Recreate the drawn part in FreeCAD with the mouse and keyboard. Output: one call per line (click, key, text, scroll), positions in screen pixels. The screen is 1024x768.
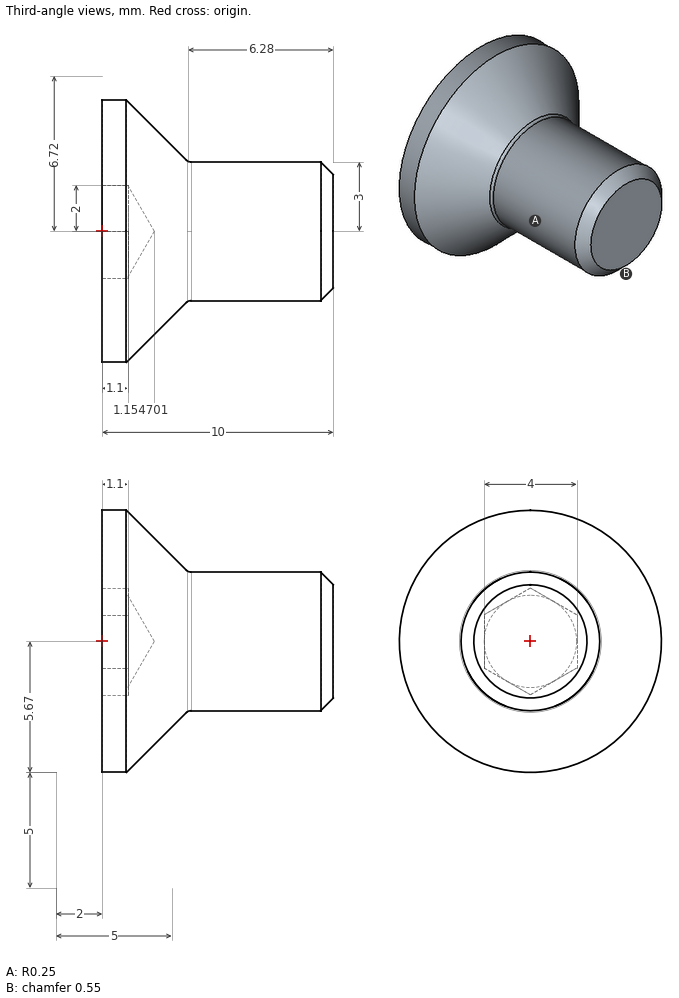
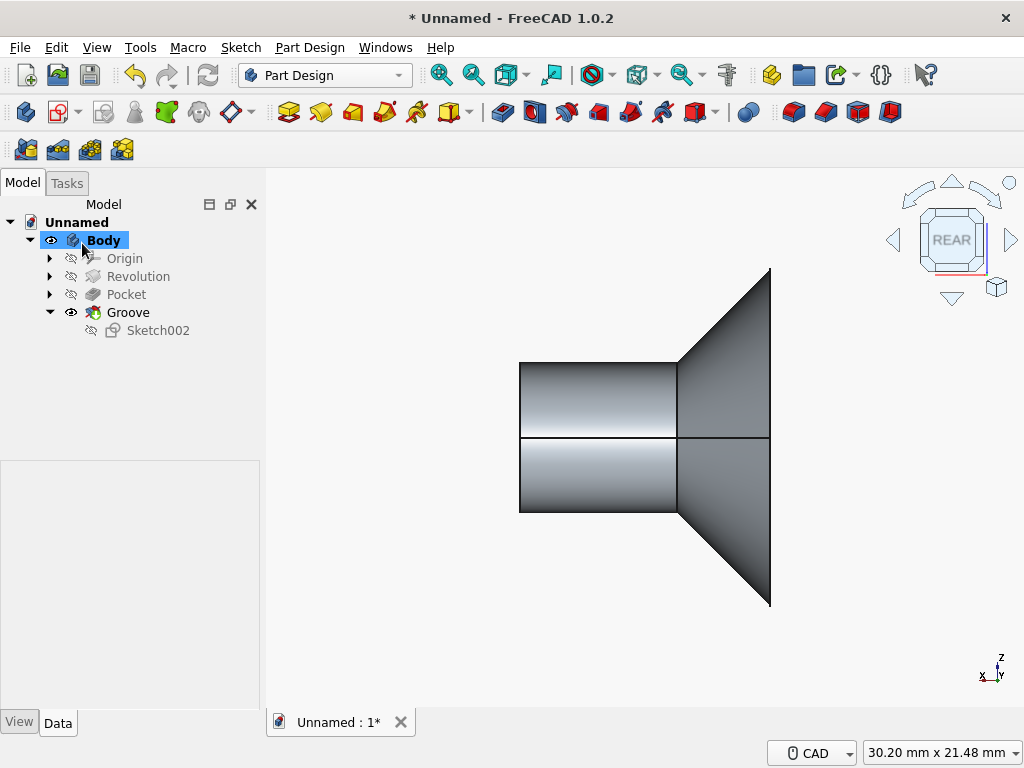
key(6)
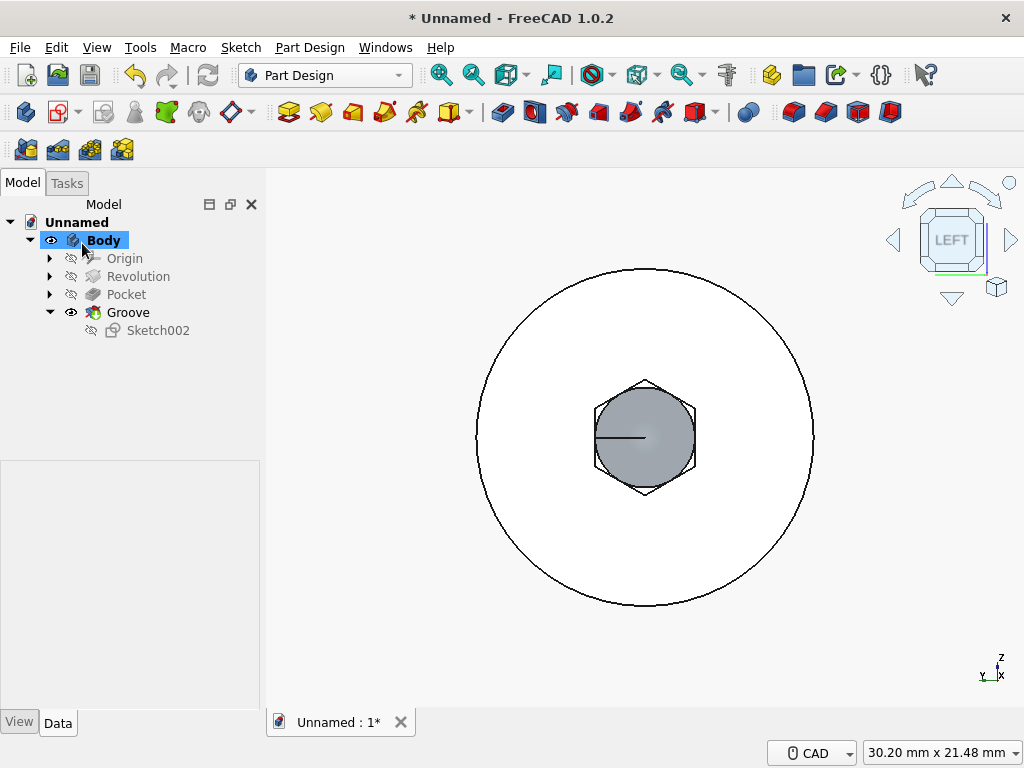
key(v)
key(3)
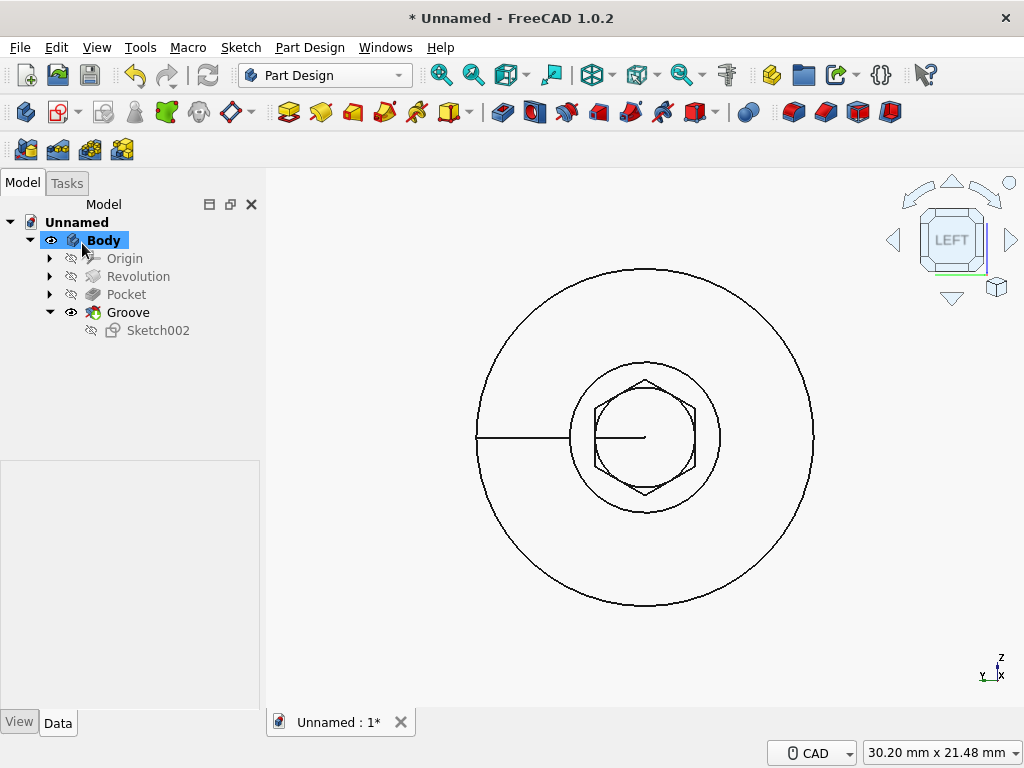
key(0)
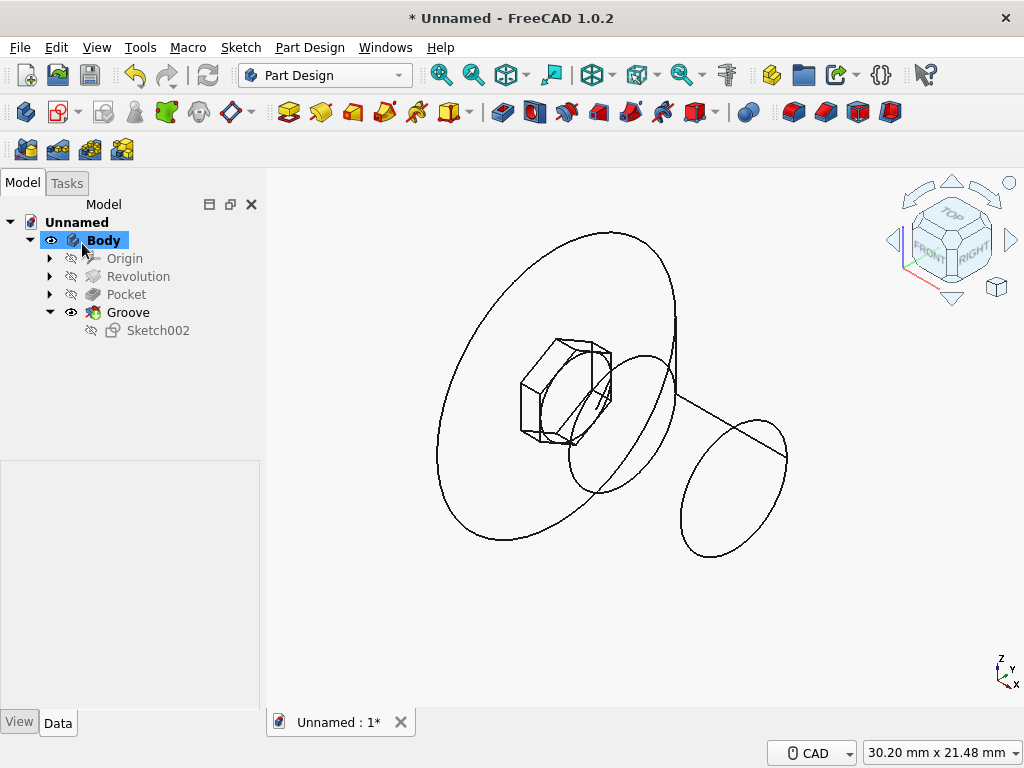
click(569, 454)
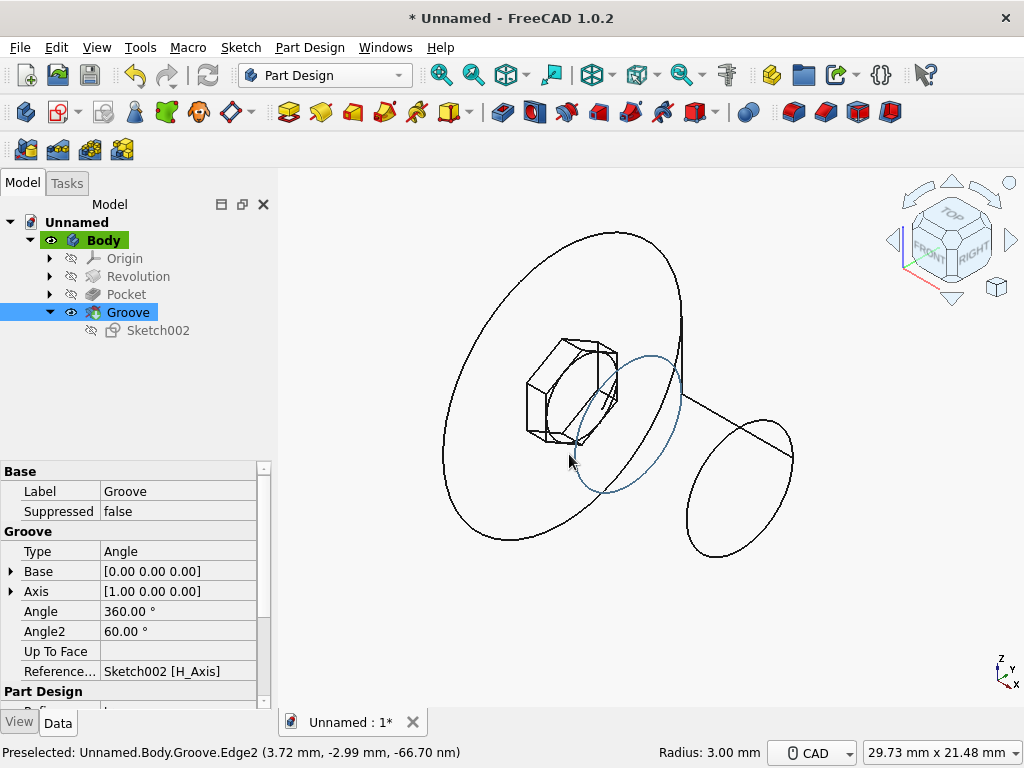
key(v)
key(1)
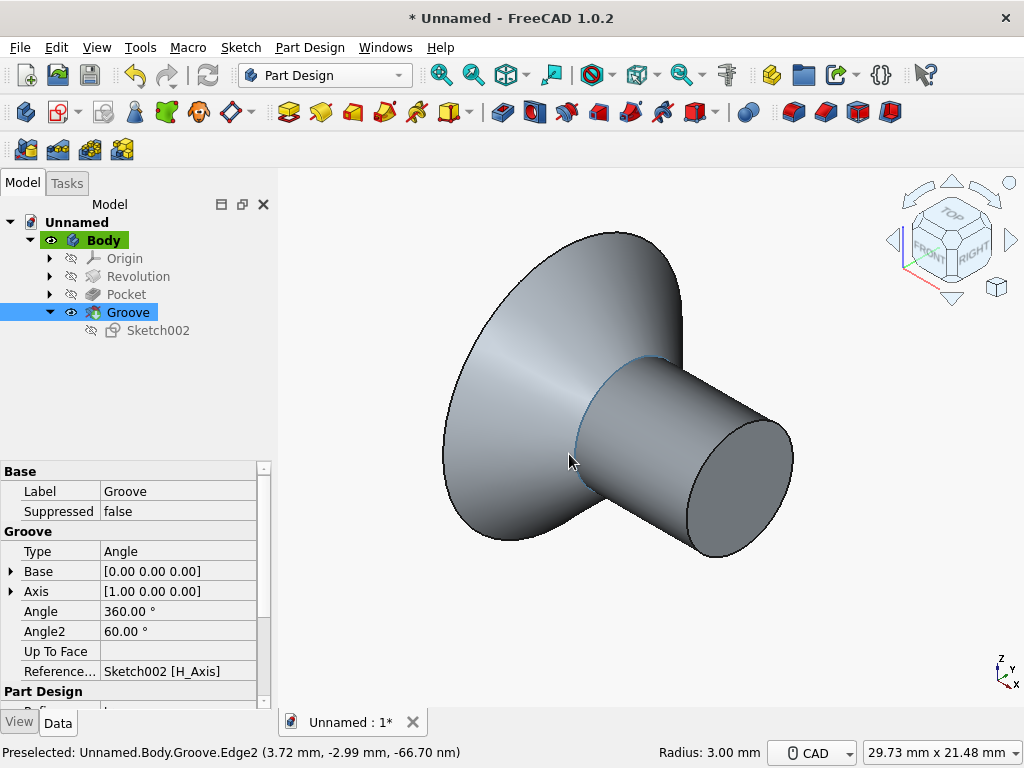
click(794, 112)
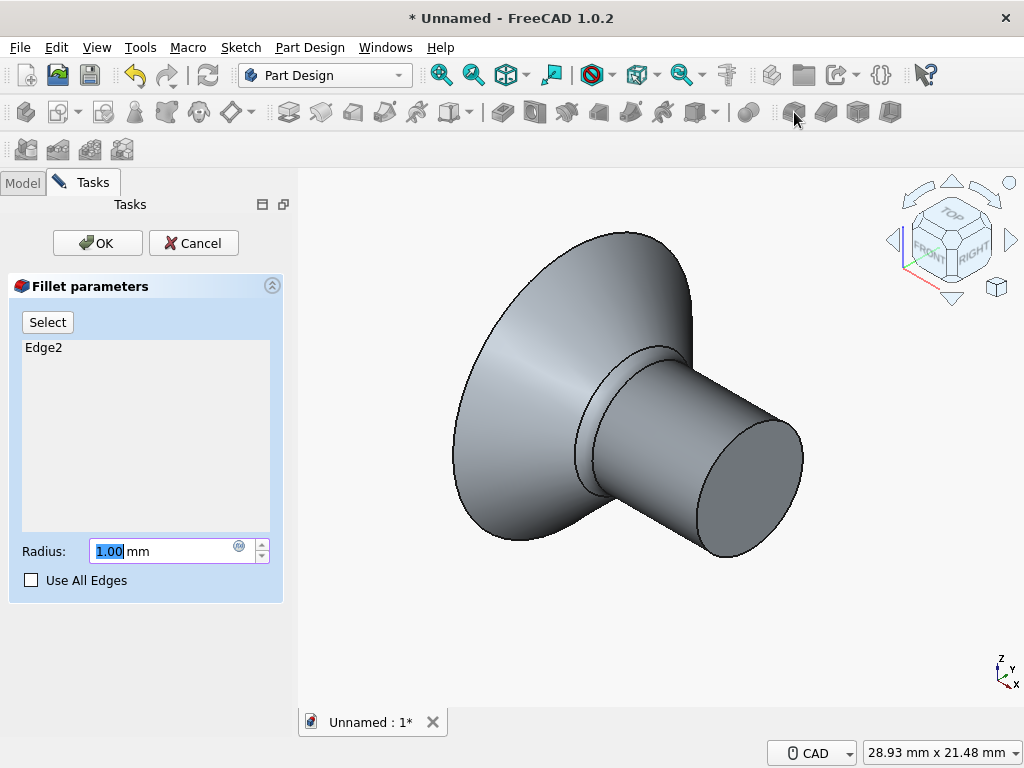
text(0.25)
key(Tab)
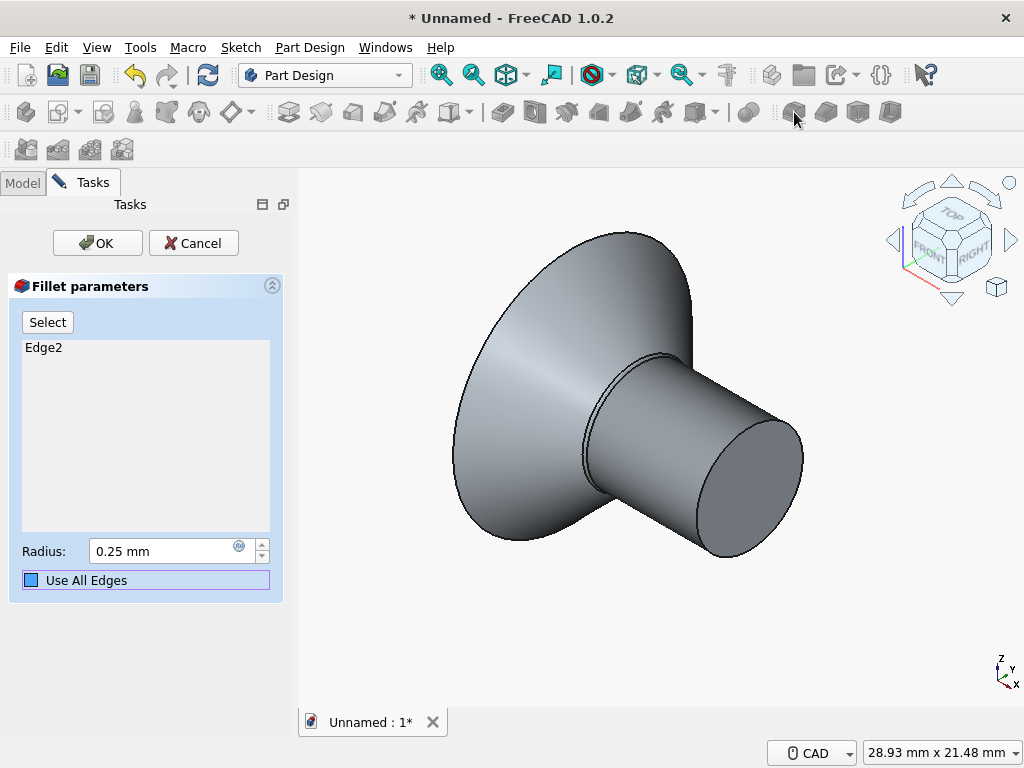
click(98, 243)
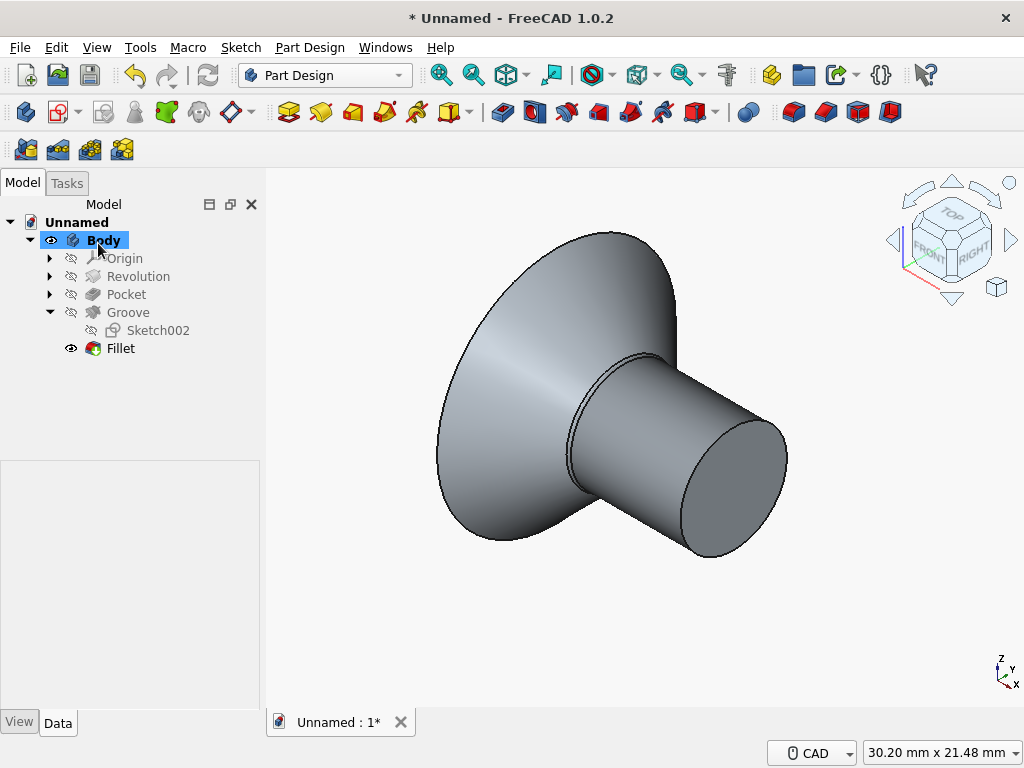
click(680, 518)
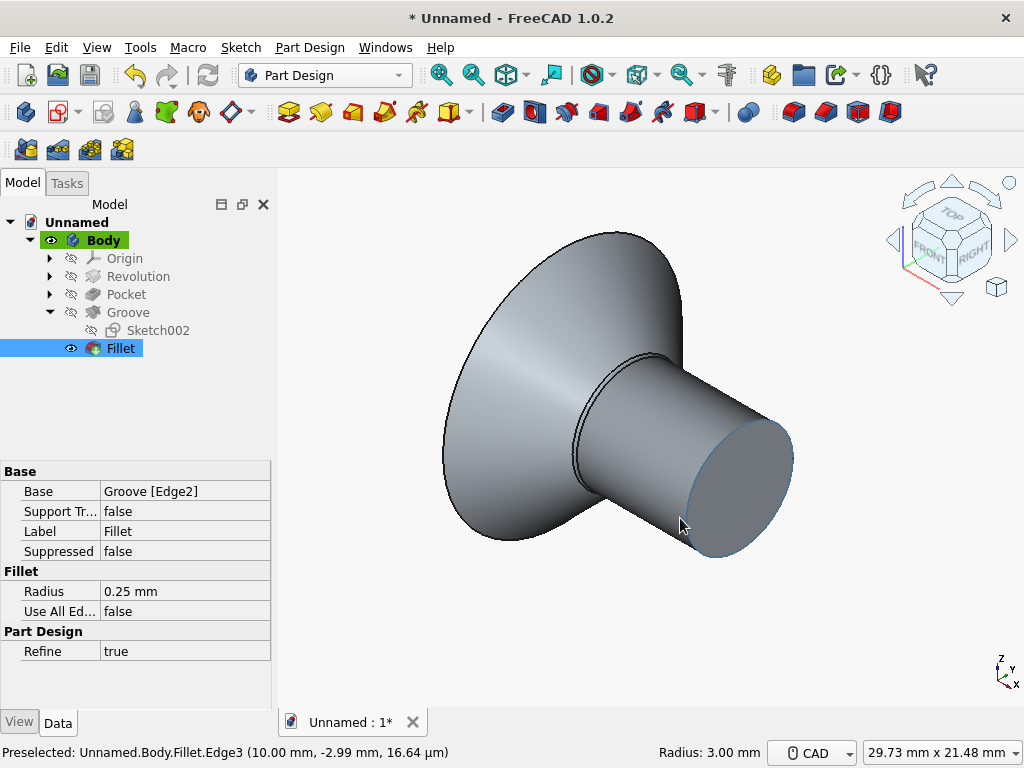
click(826, 112)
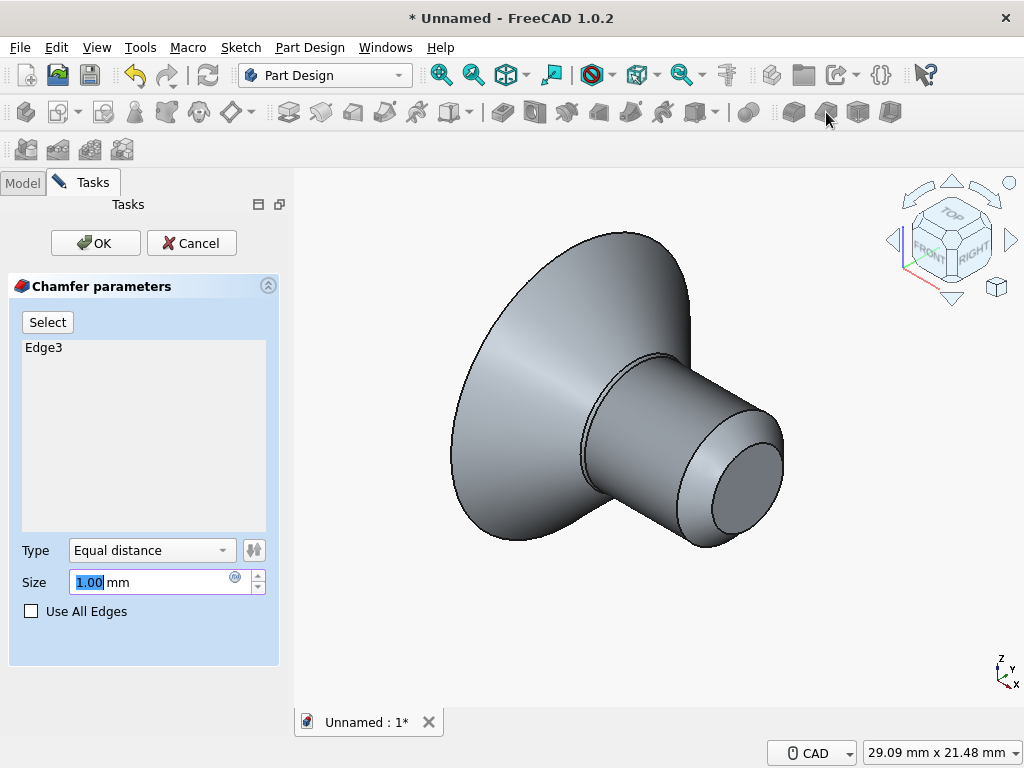
text(0.55)
key(Tab)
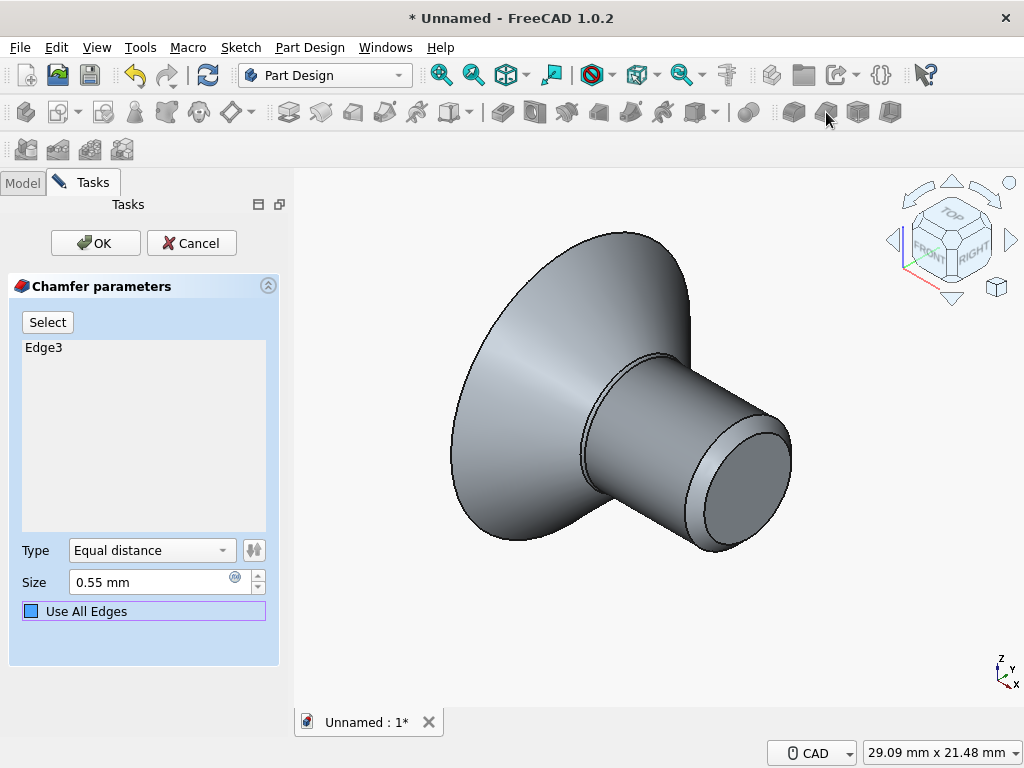
click(96, 243)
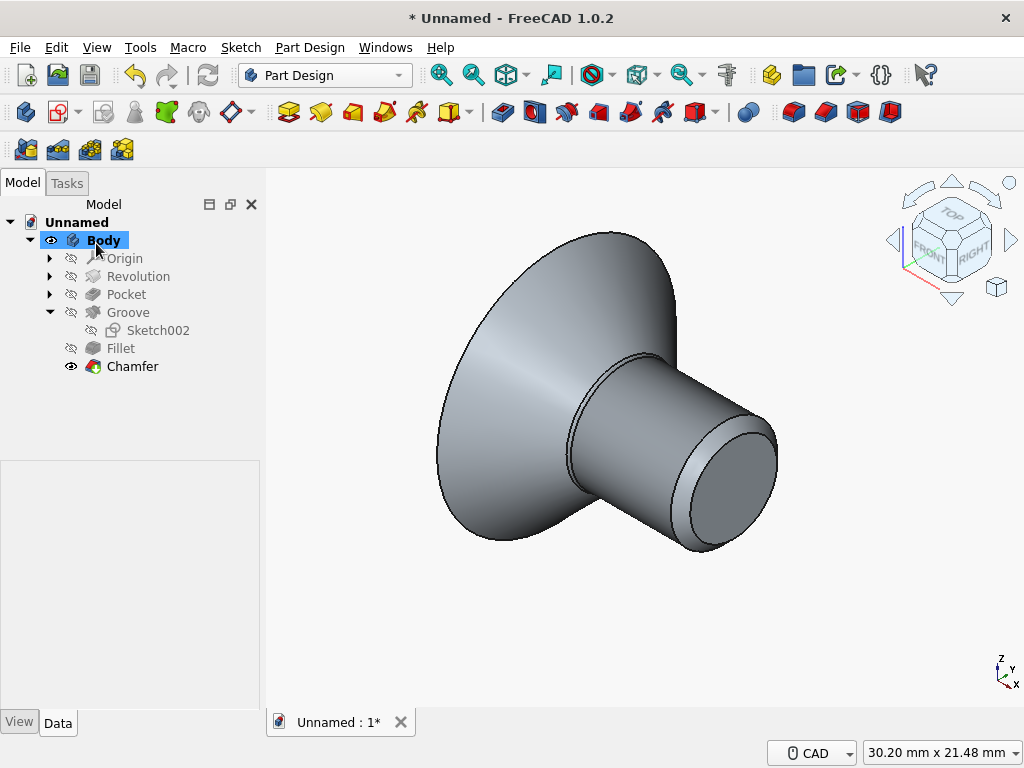
click(58, 112)